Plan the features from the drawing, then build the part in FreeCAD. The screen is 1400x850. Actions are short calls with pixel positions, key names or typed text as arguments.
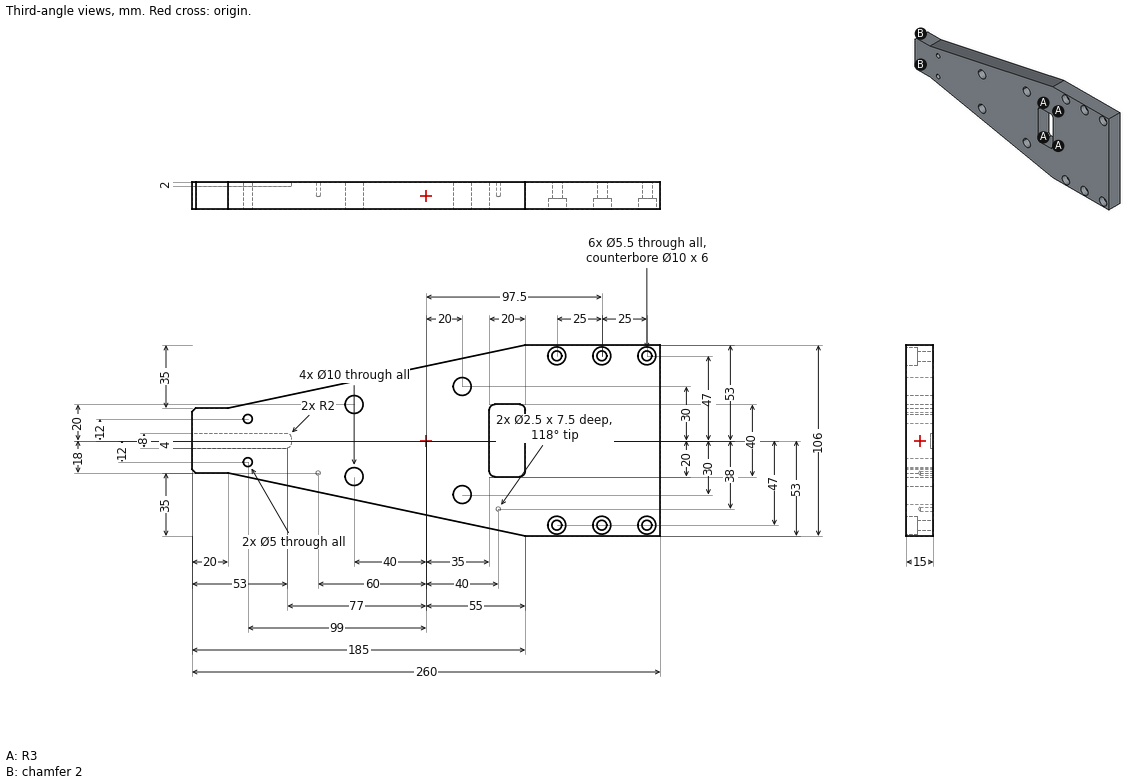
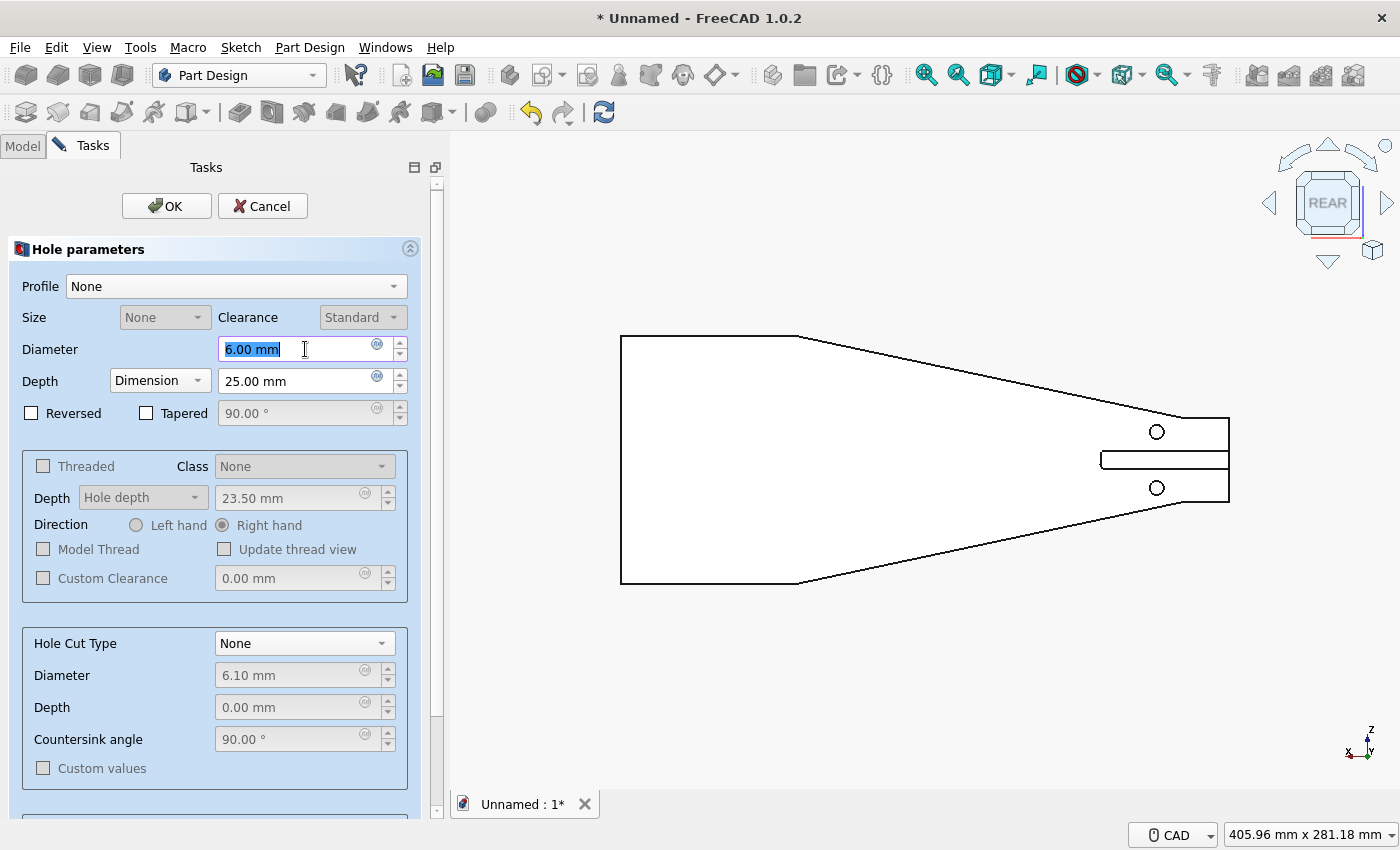
text(5)
key(Tab)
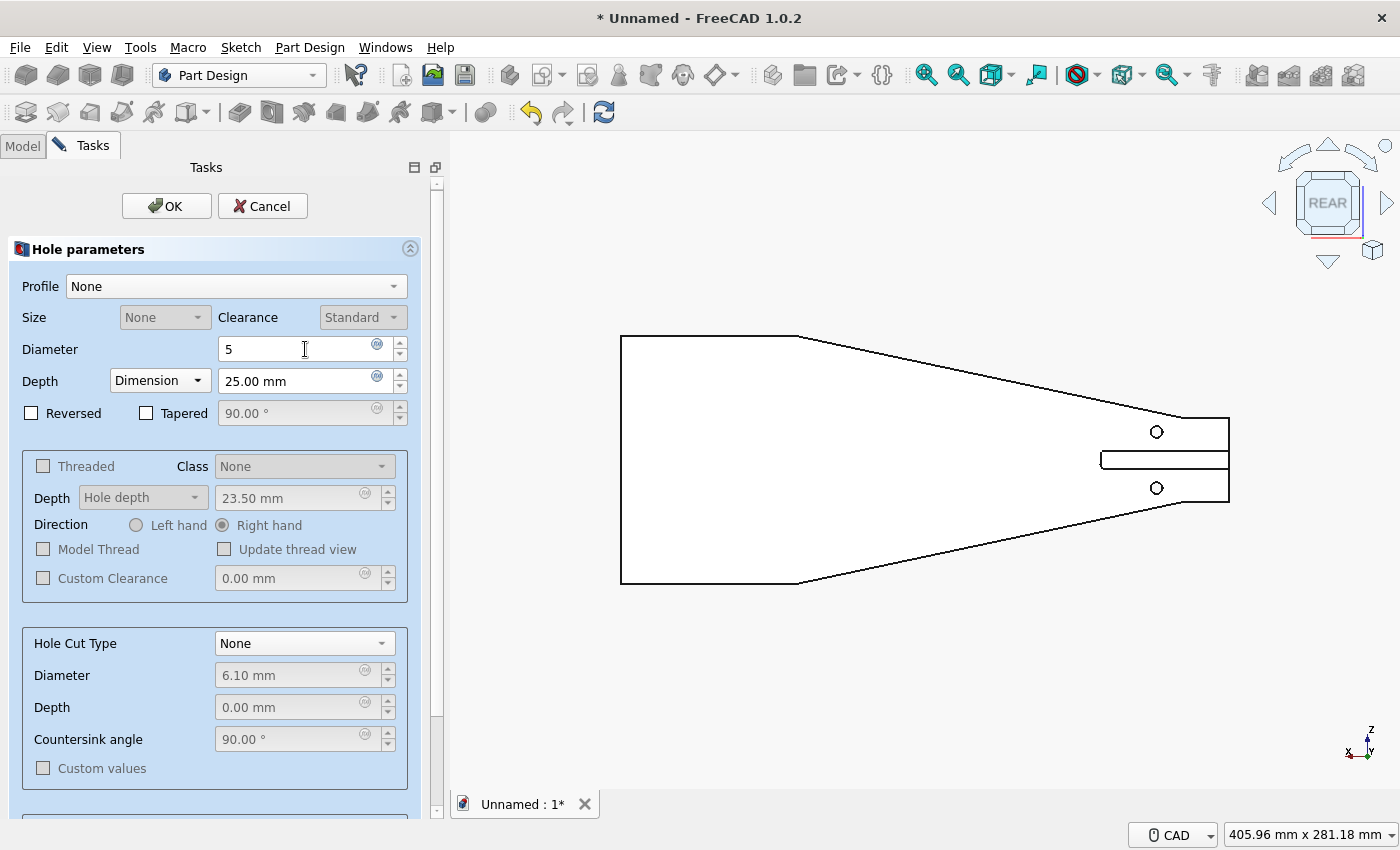
click(161, 380)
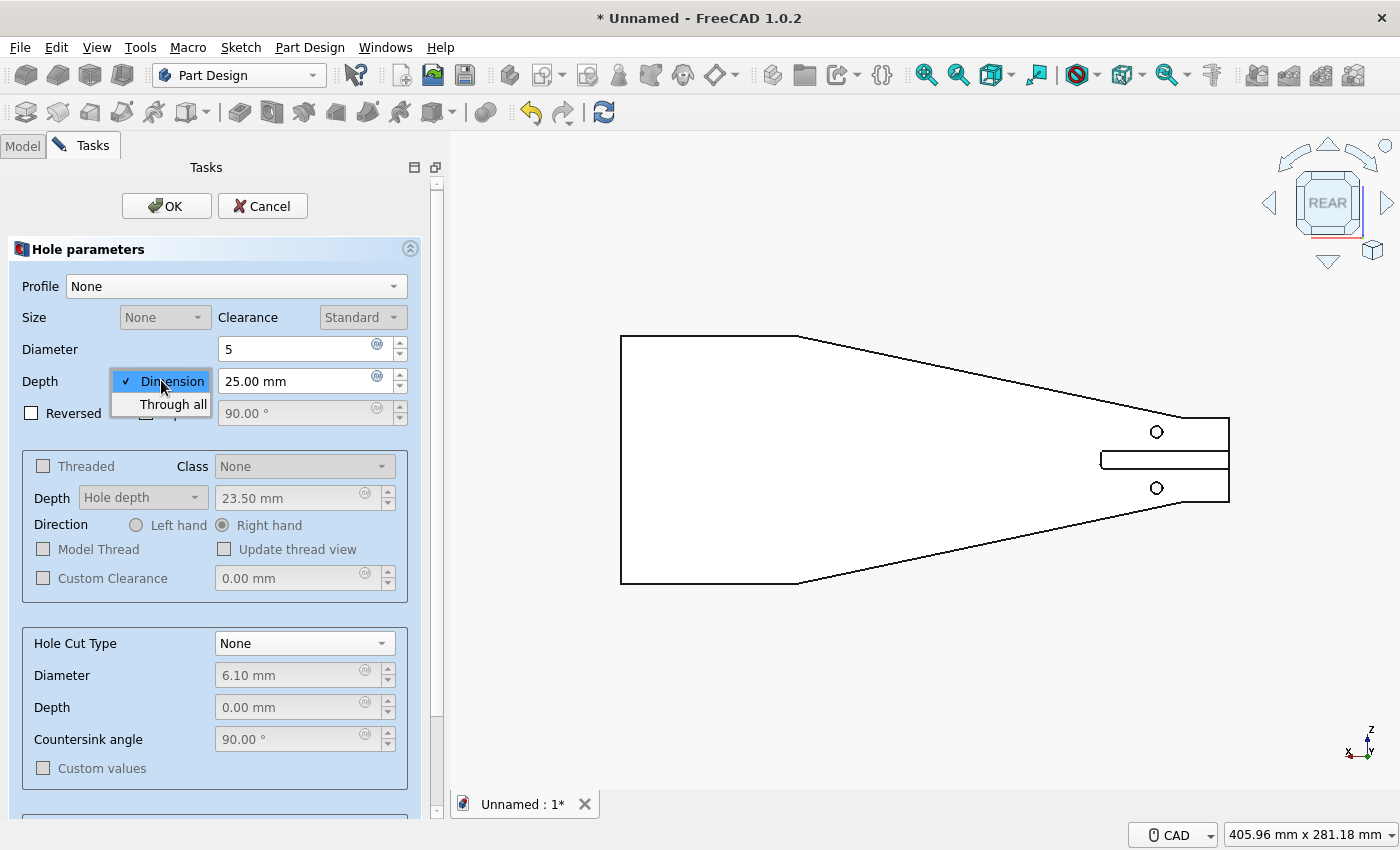
click(160, 404)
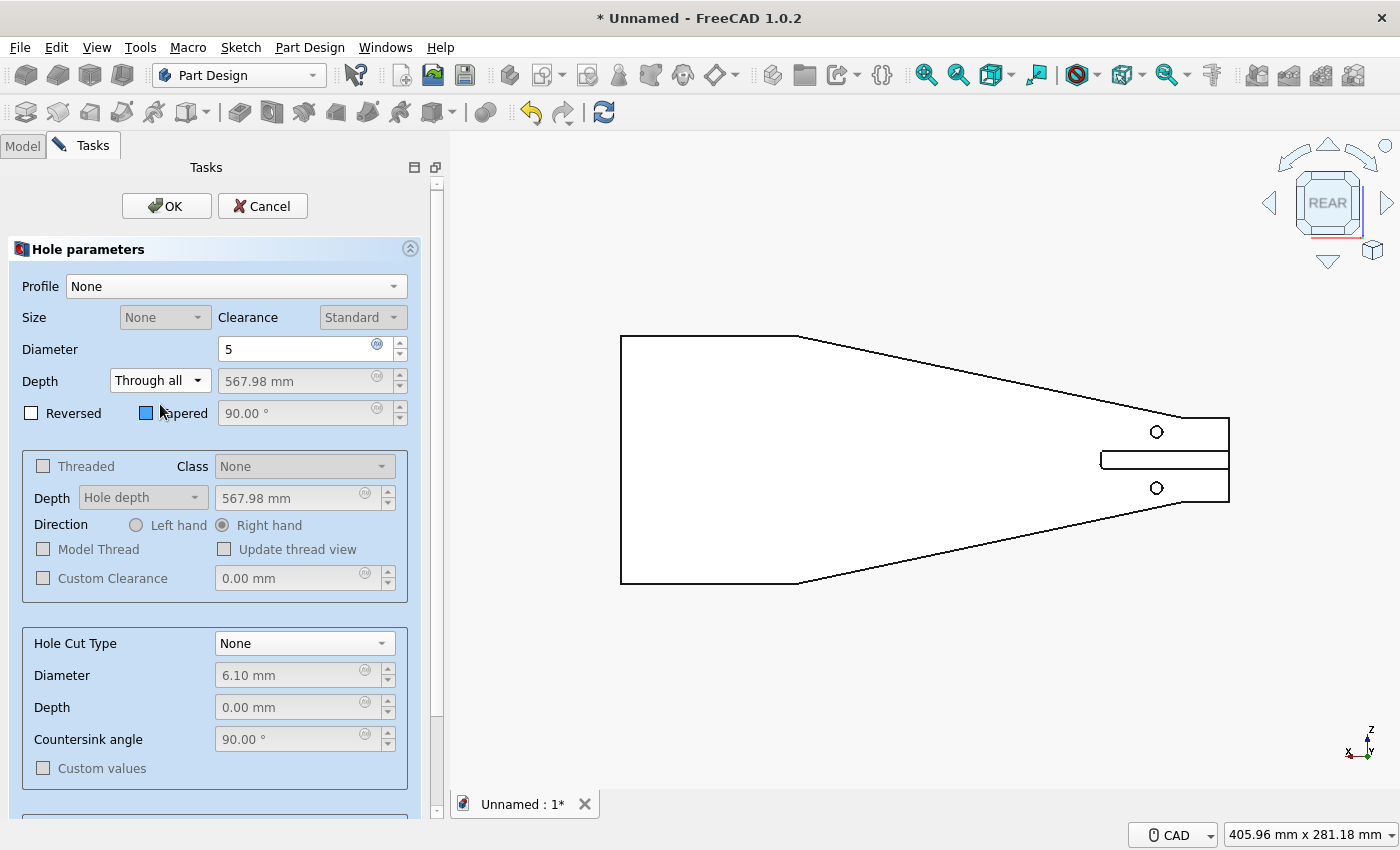
click(167, 206)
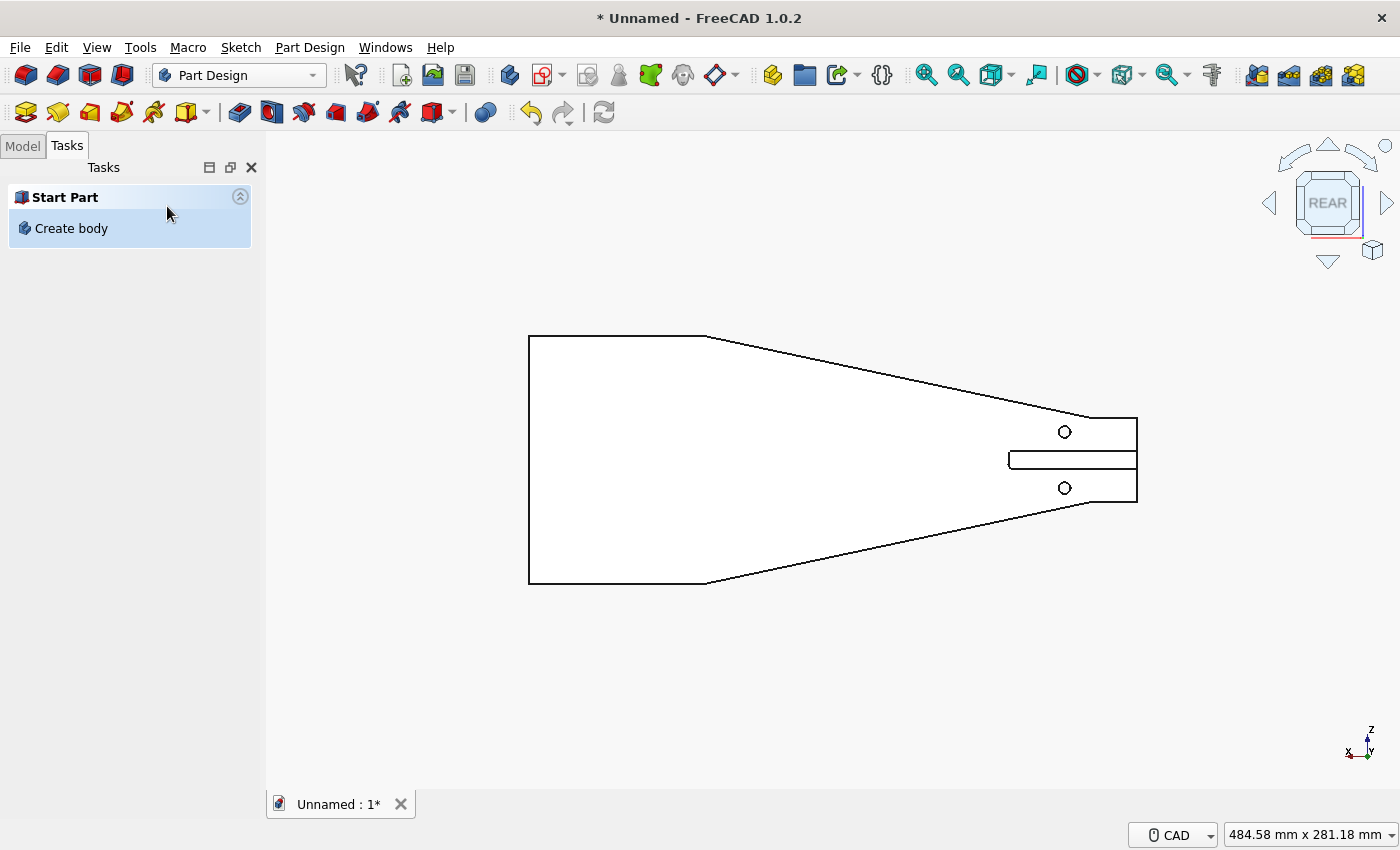
click(659, 459)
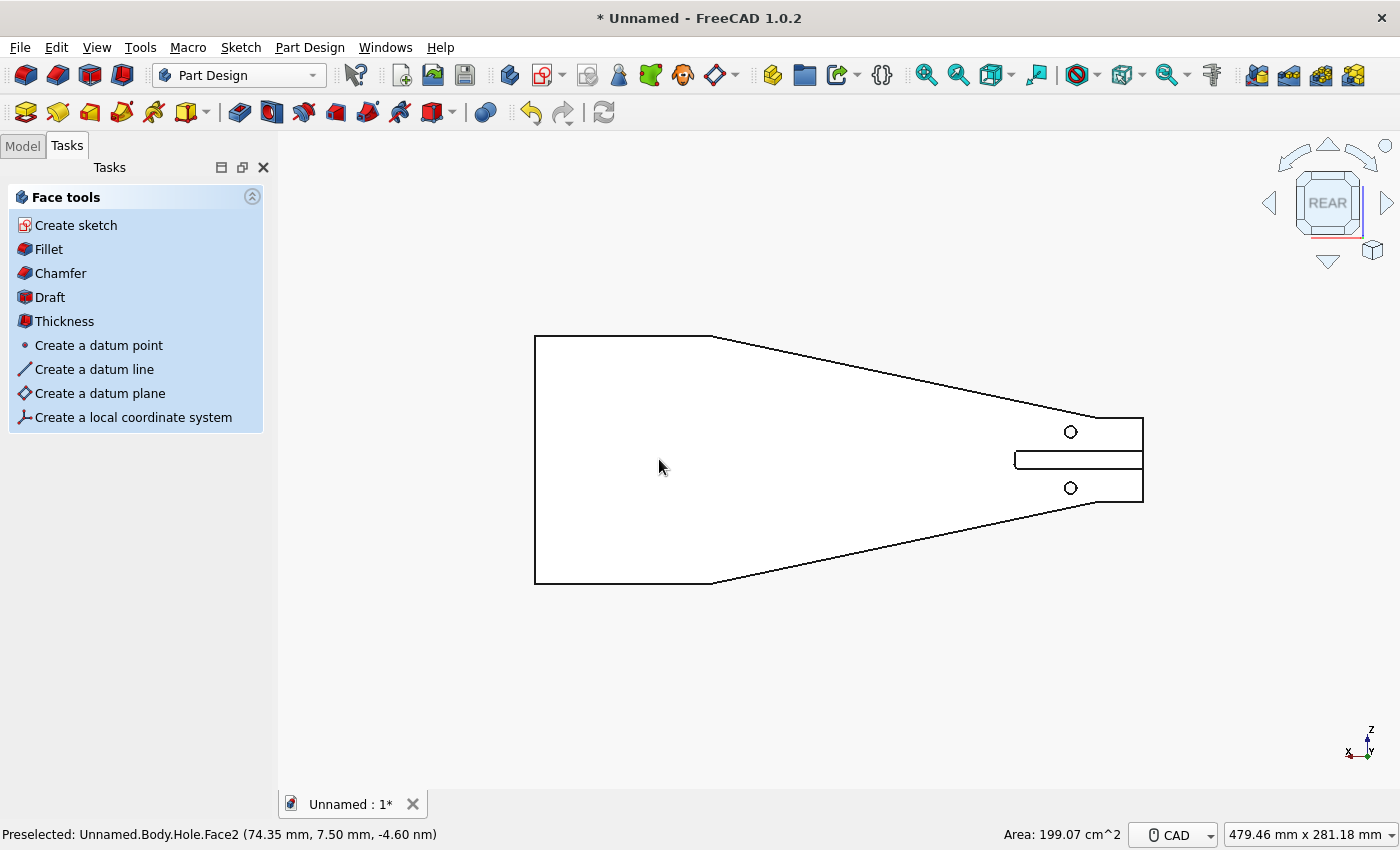
click(542, 76)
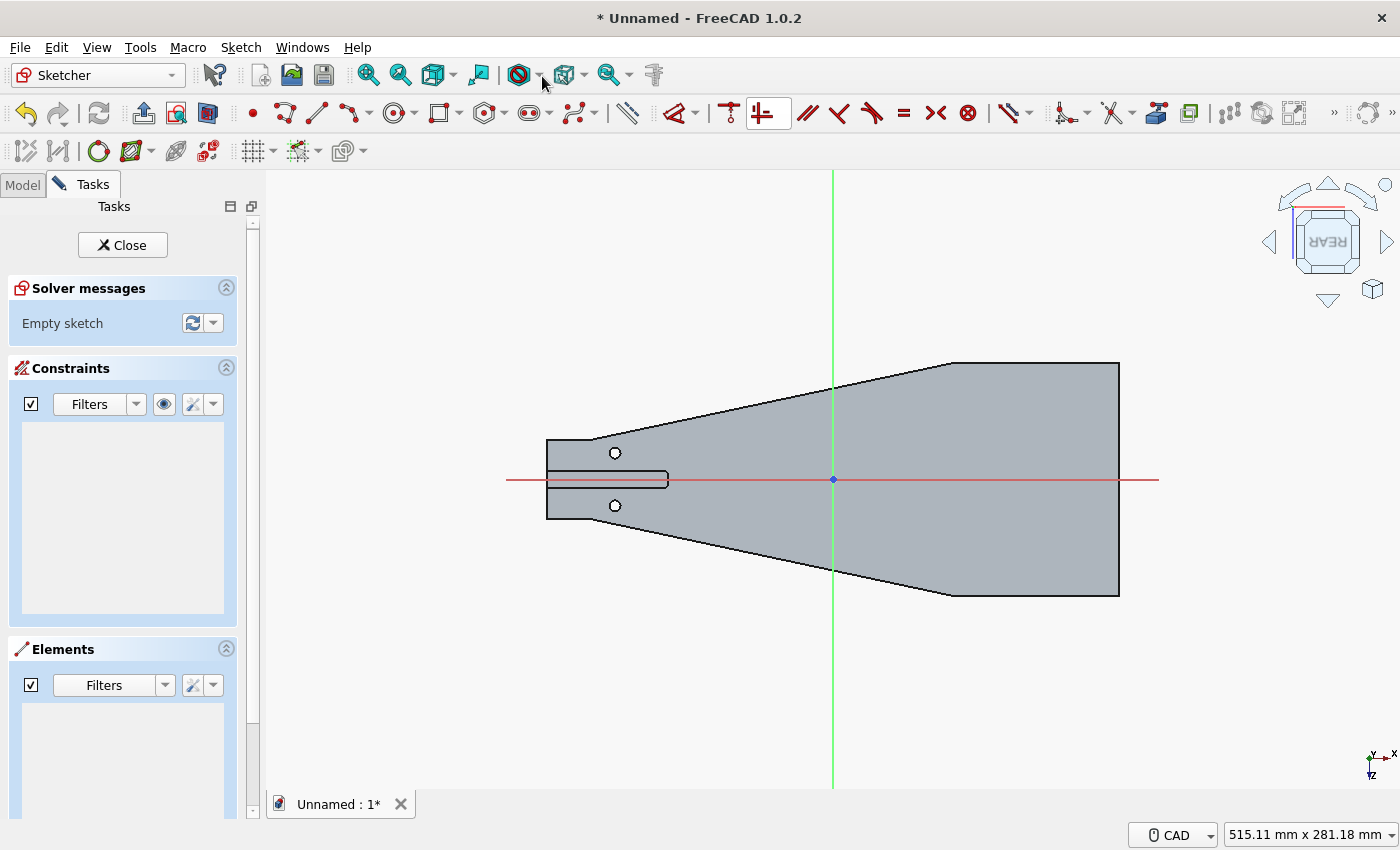
scroll(926, 479, up, 8)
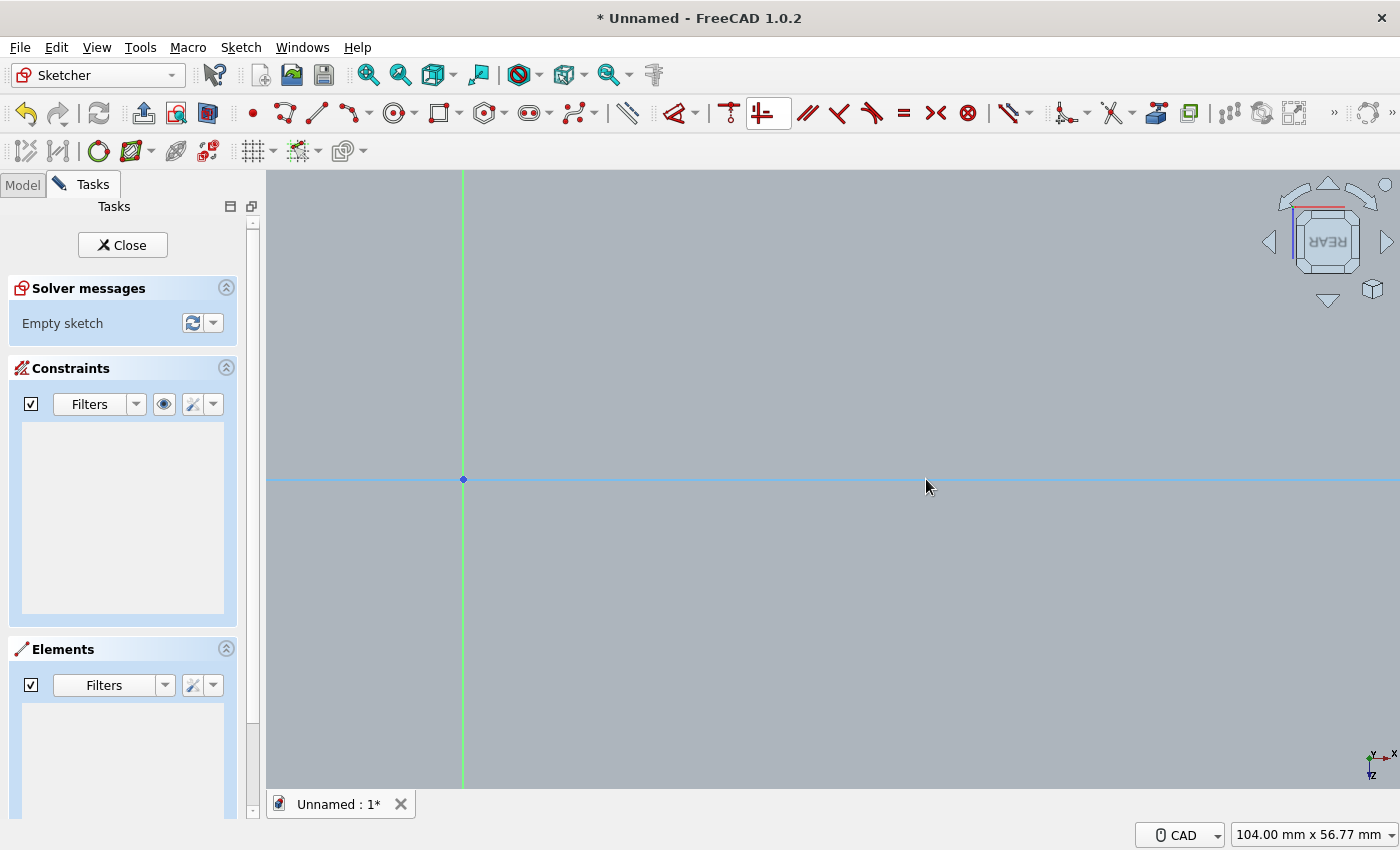
click(440, 114)